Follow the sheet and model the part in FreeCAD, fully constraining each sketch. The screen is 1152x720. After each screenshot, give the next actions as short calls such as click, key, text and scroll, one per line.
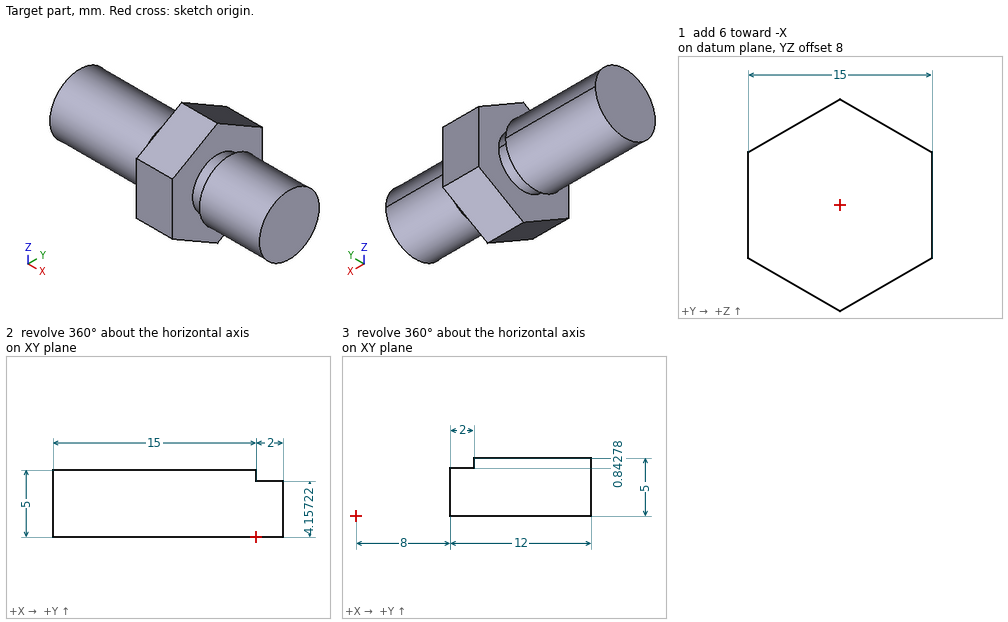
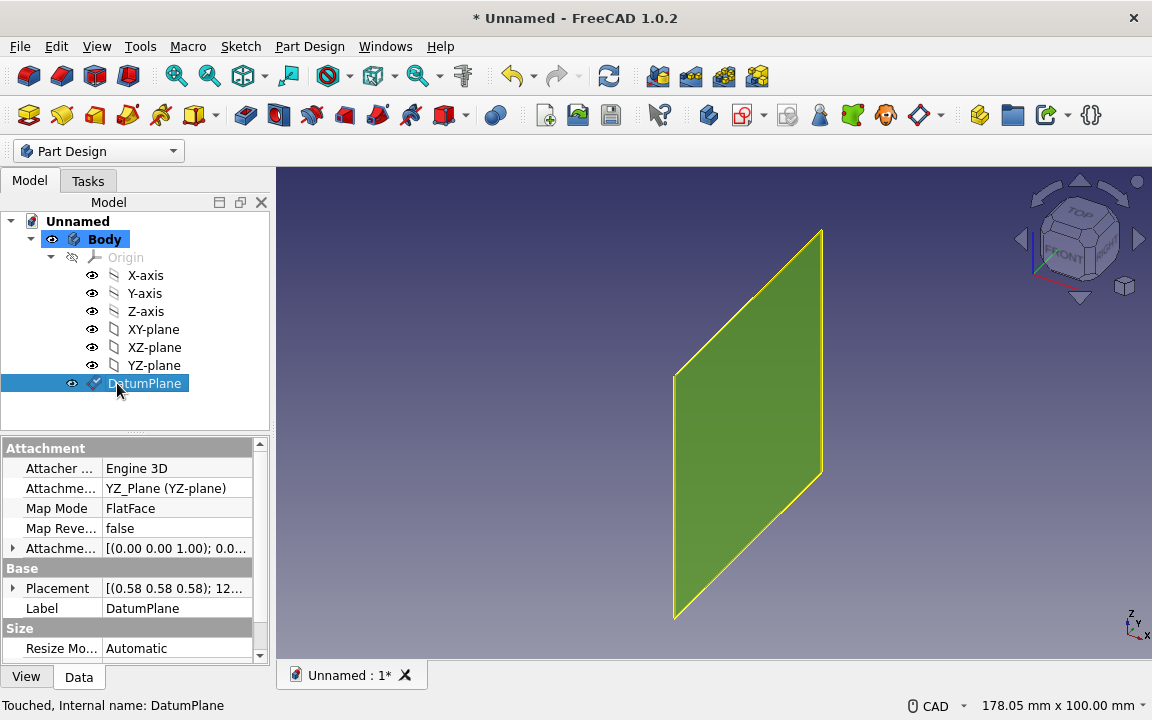
click(742, 116)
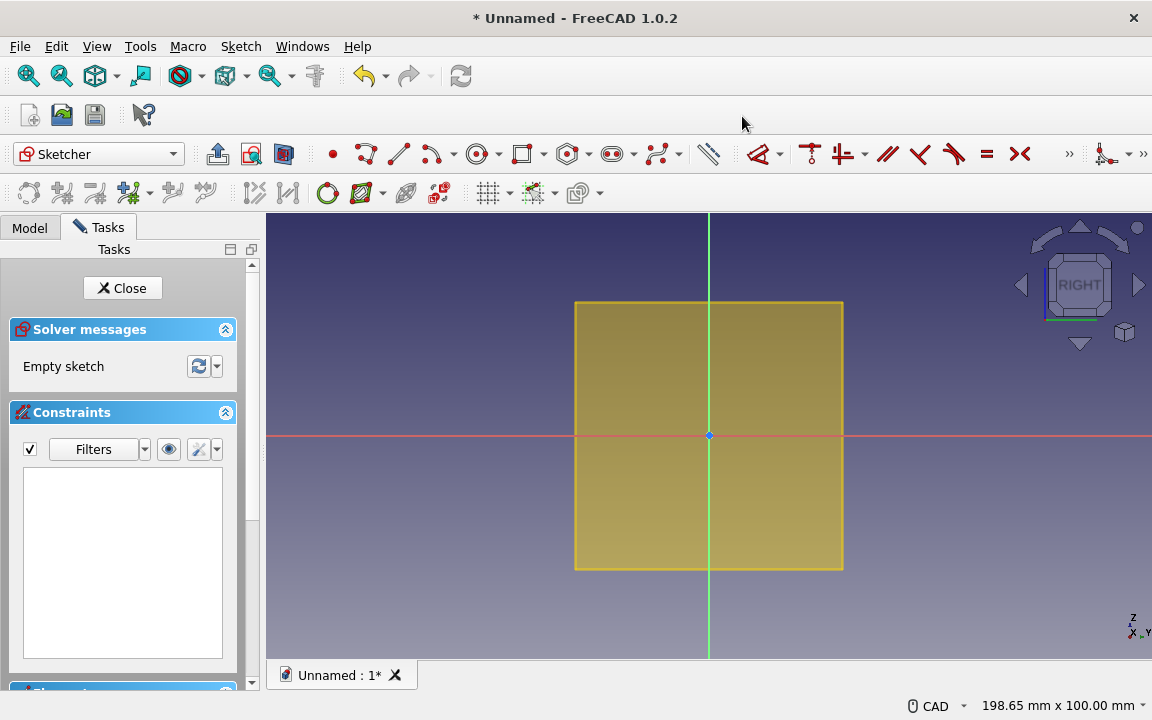
scroll(739, 436, up, 6)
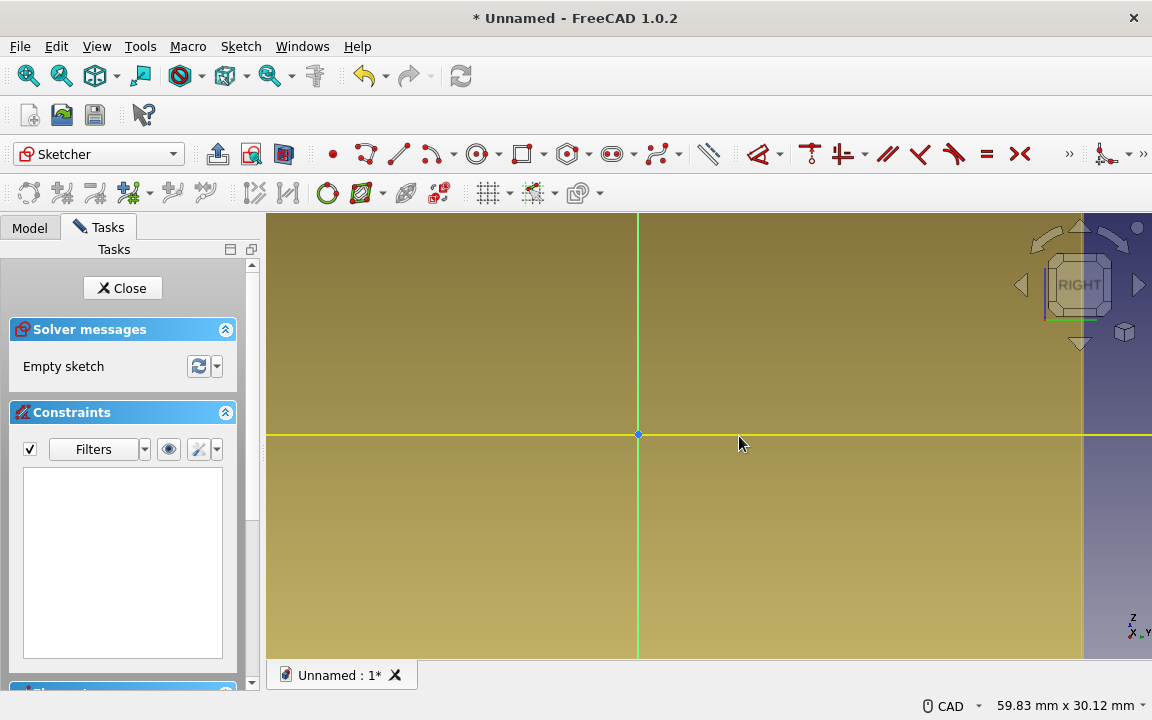
click(566, 154)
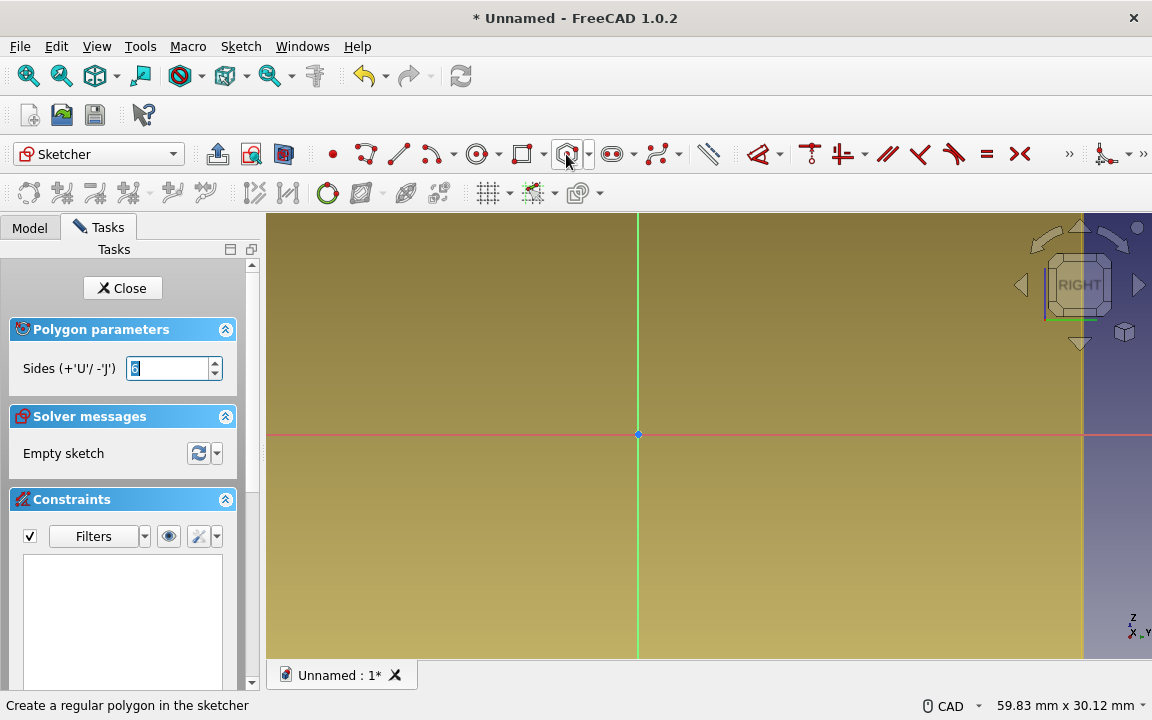
click(638, 435)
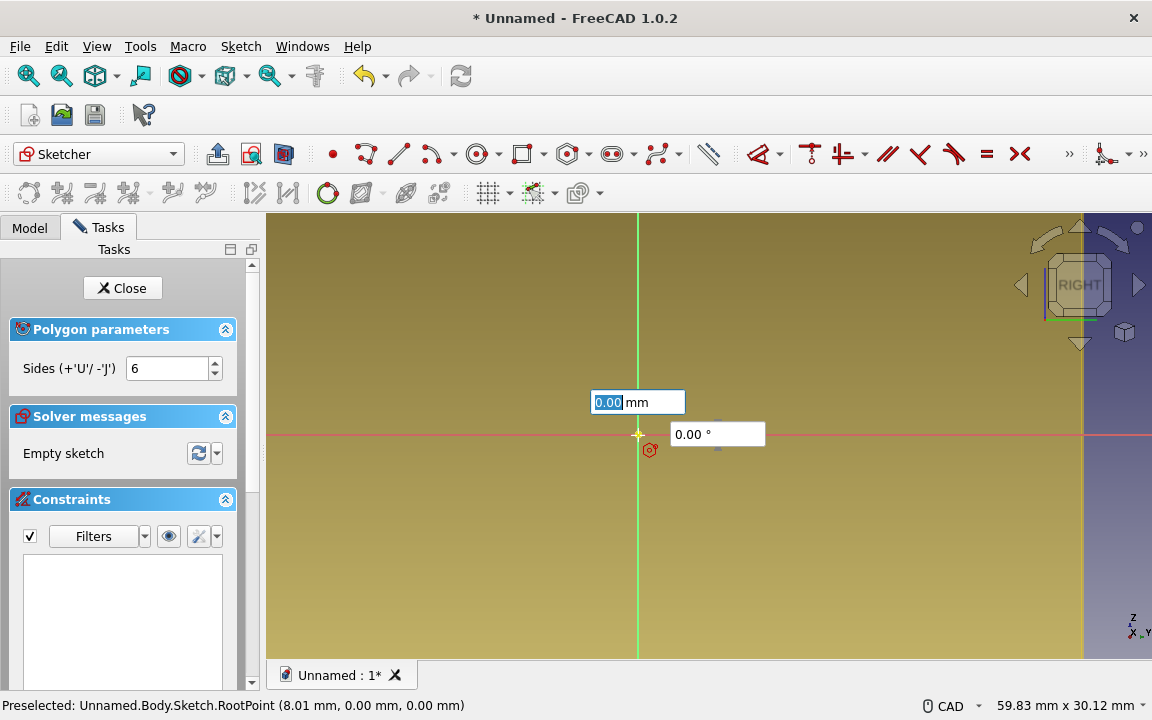
click(638, 307)
right_click(638, 307)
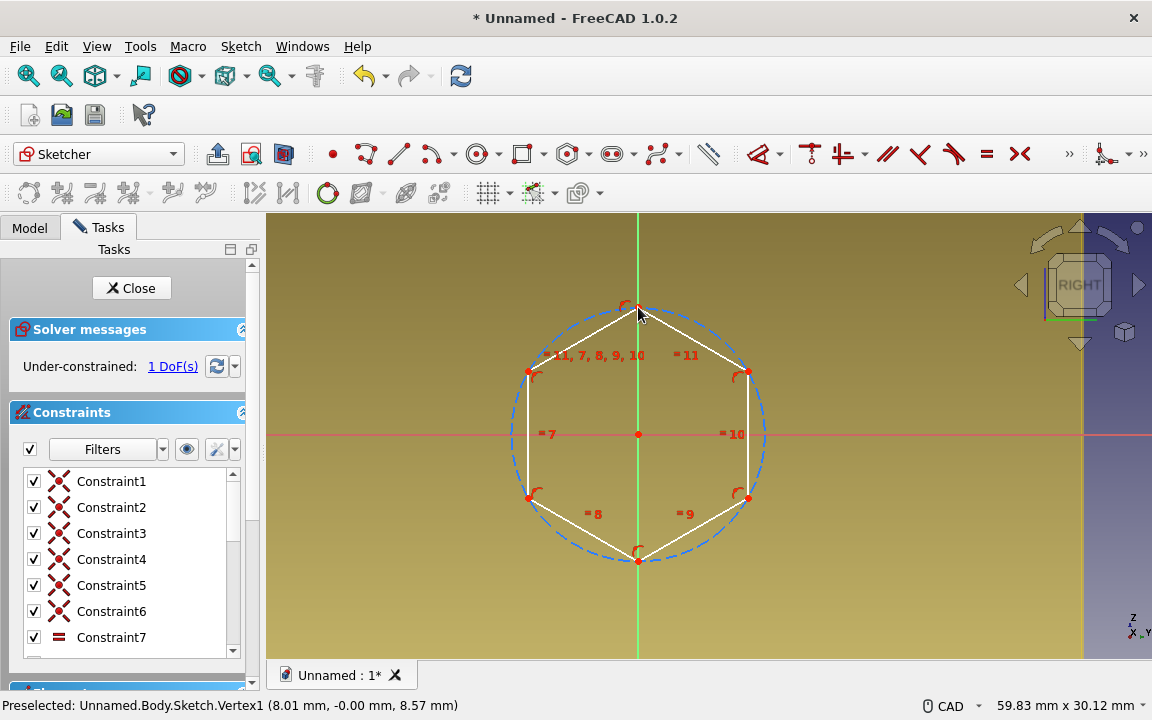
click(528, 371)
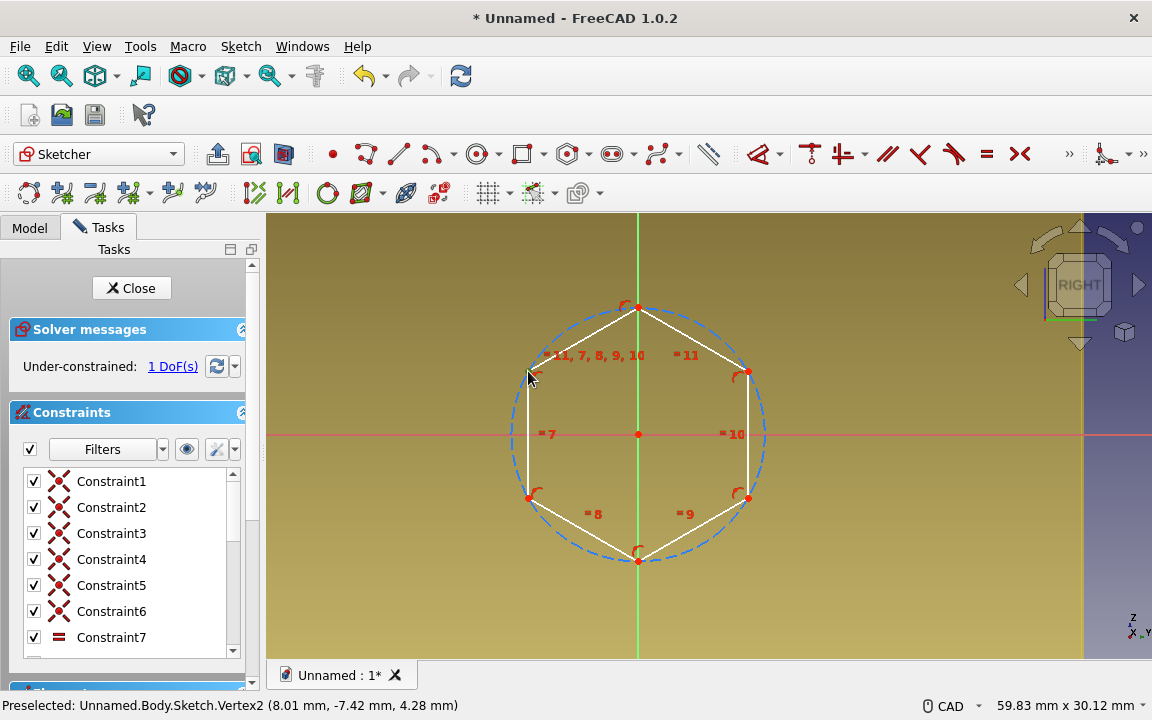
click(748, 498)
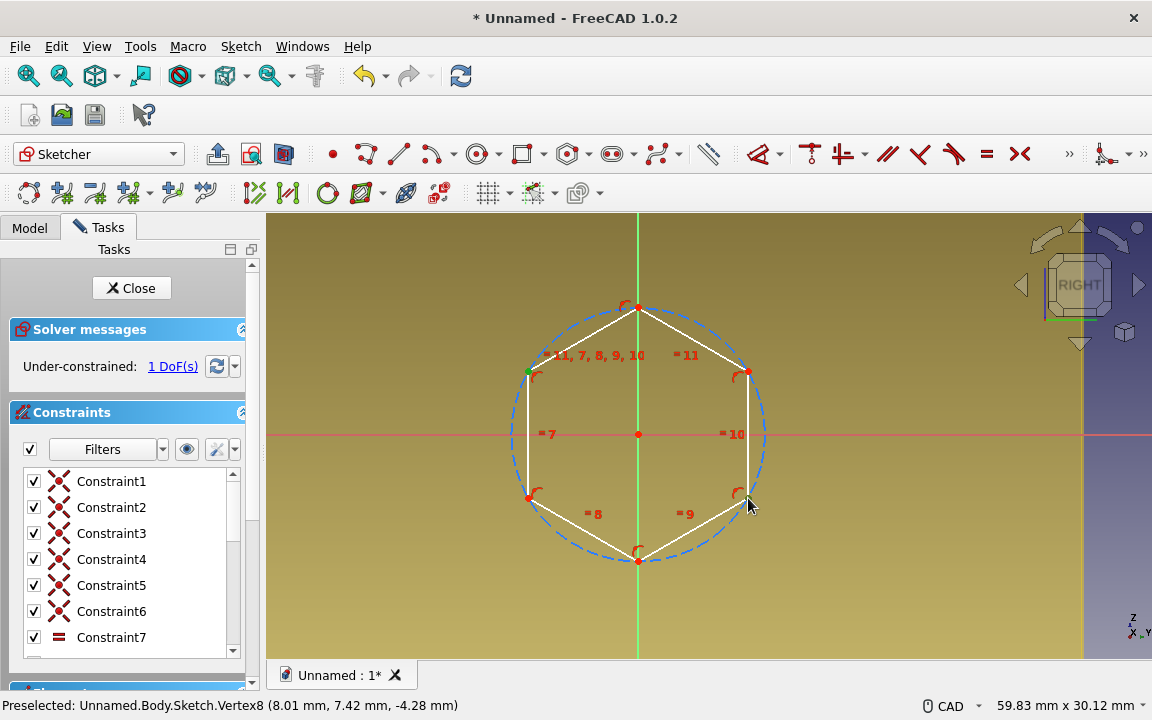
key(l)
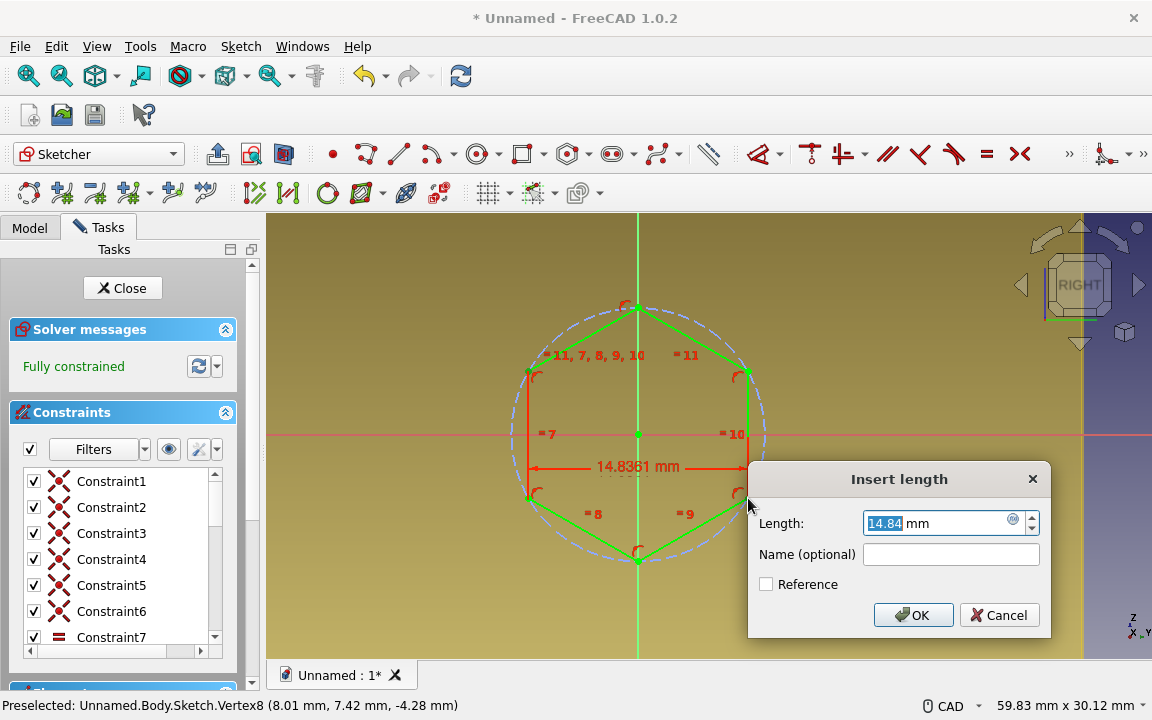
text(15)
key(Return)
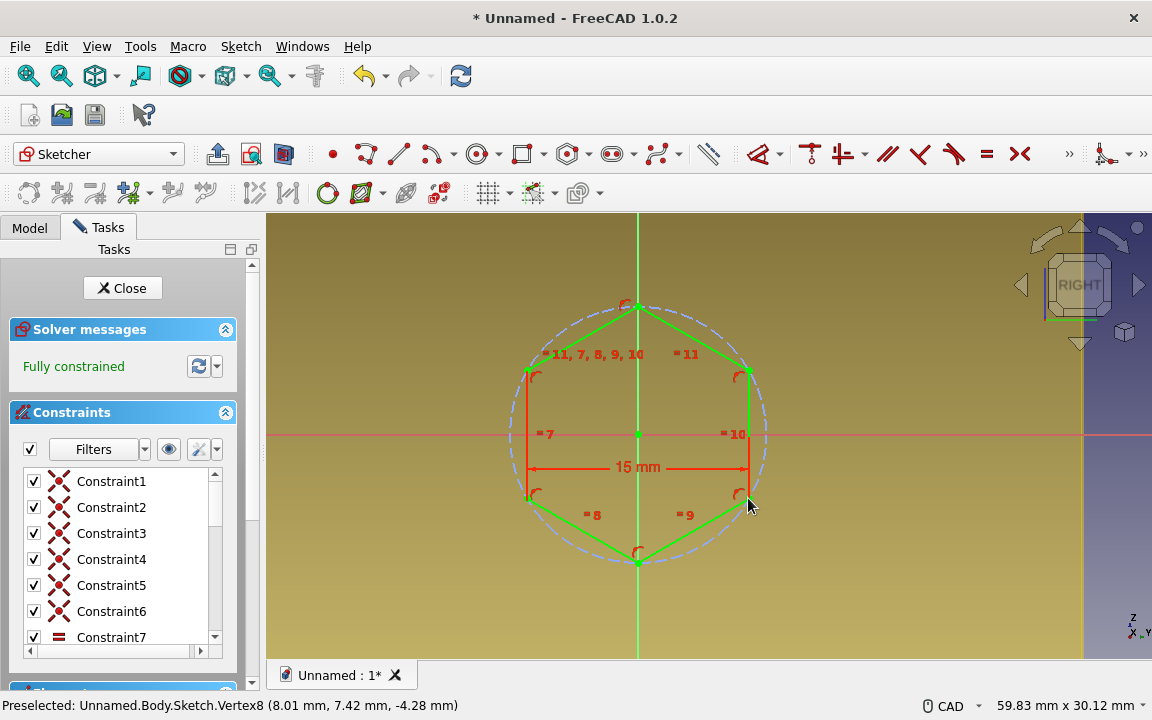
click(123, 288)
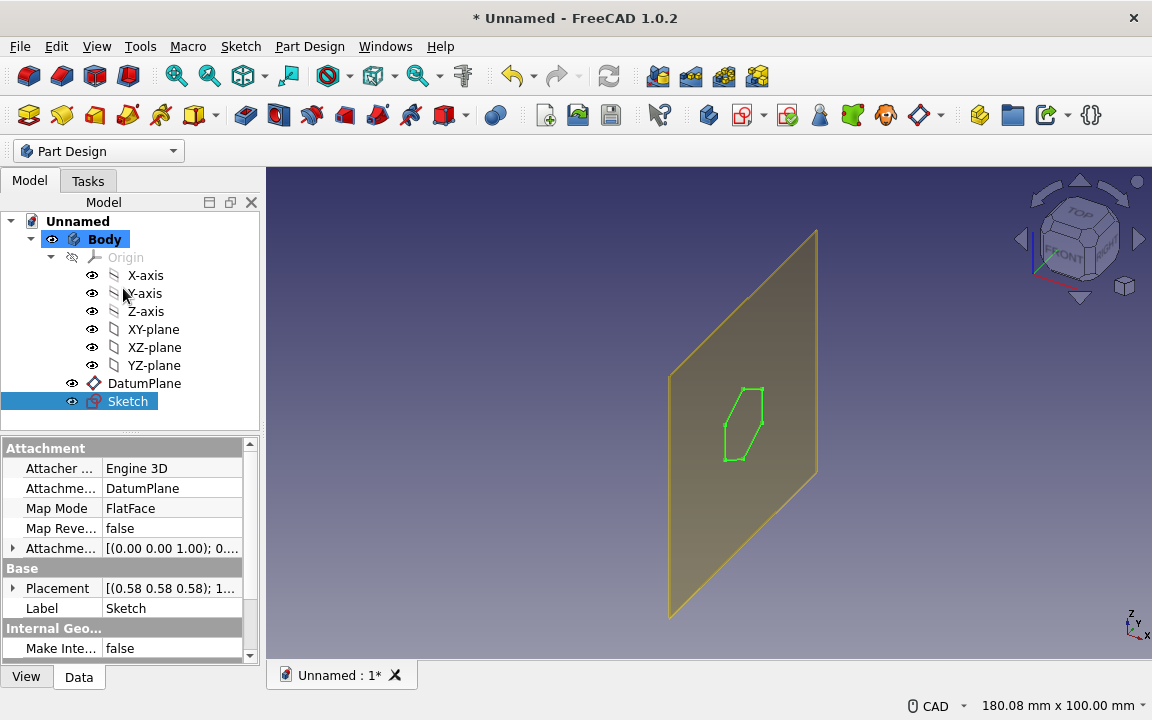
click(29, 116)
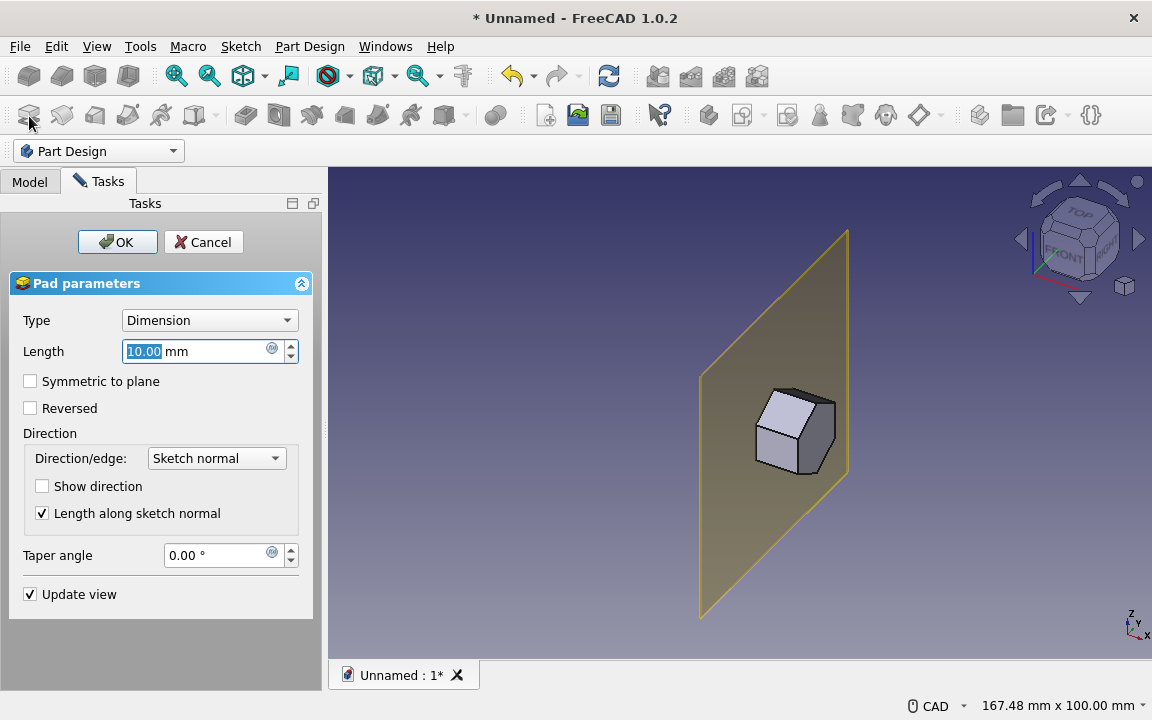
text(6)
key(Tab)